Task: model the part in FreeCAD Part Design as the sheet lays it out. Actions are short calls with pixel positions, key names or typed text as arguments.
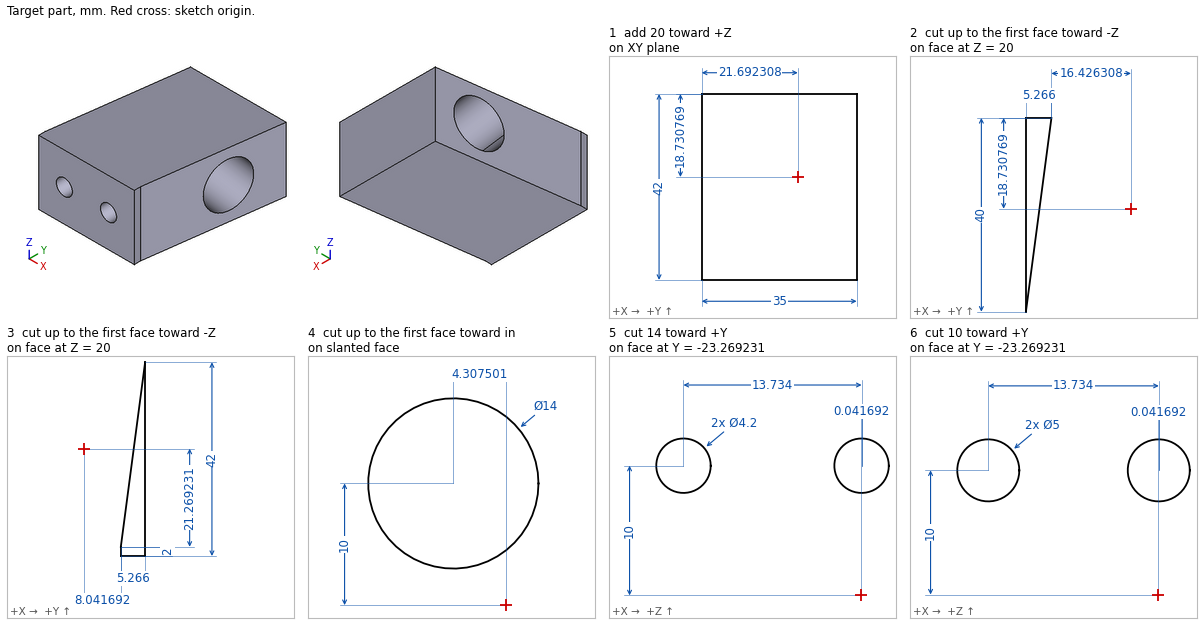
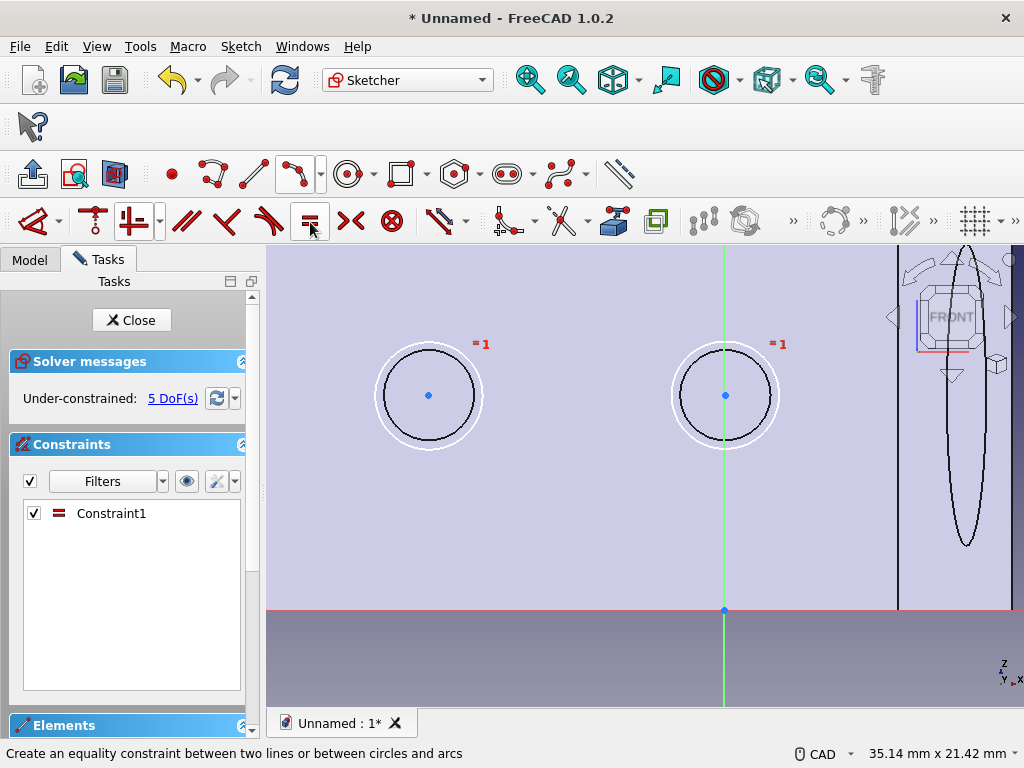
click(429, 396)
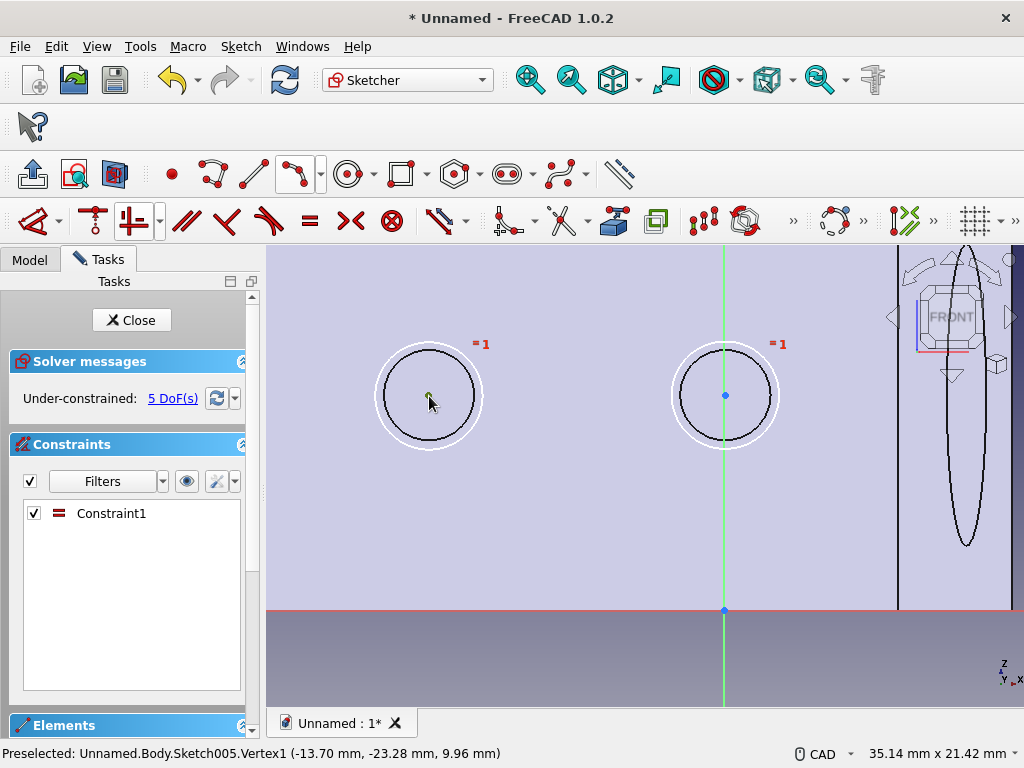
click(725, 395)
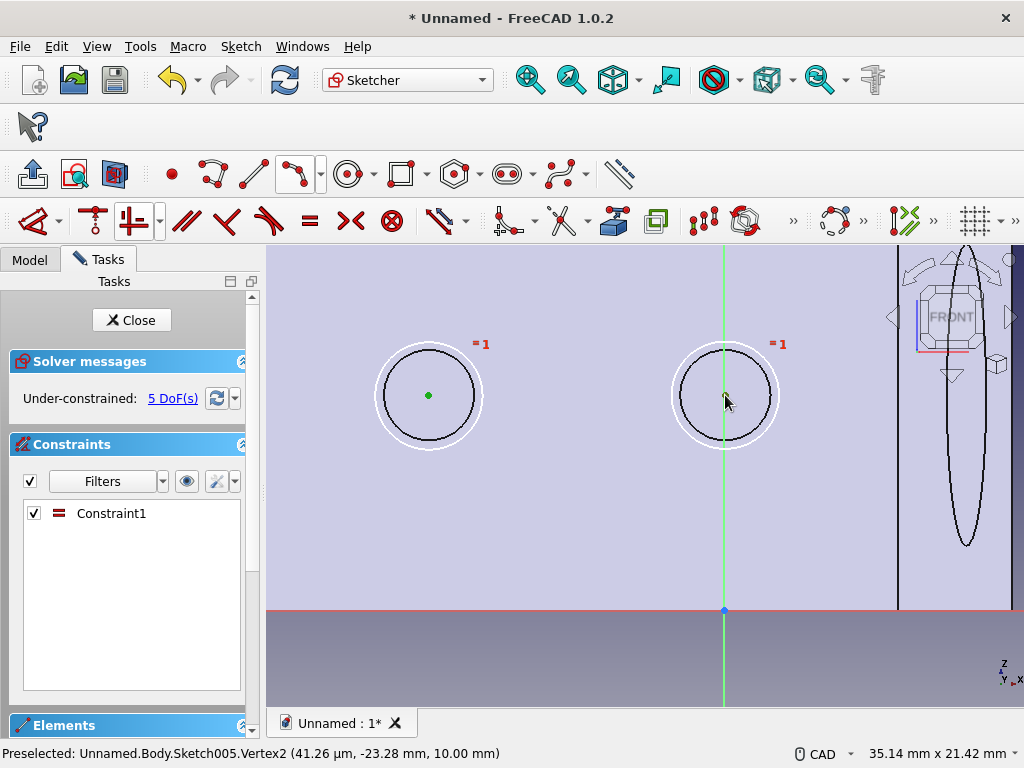
click(160, 222)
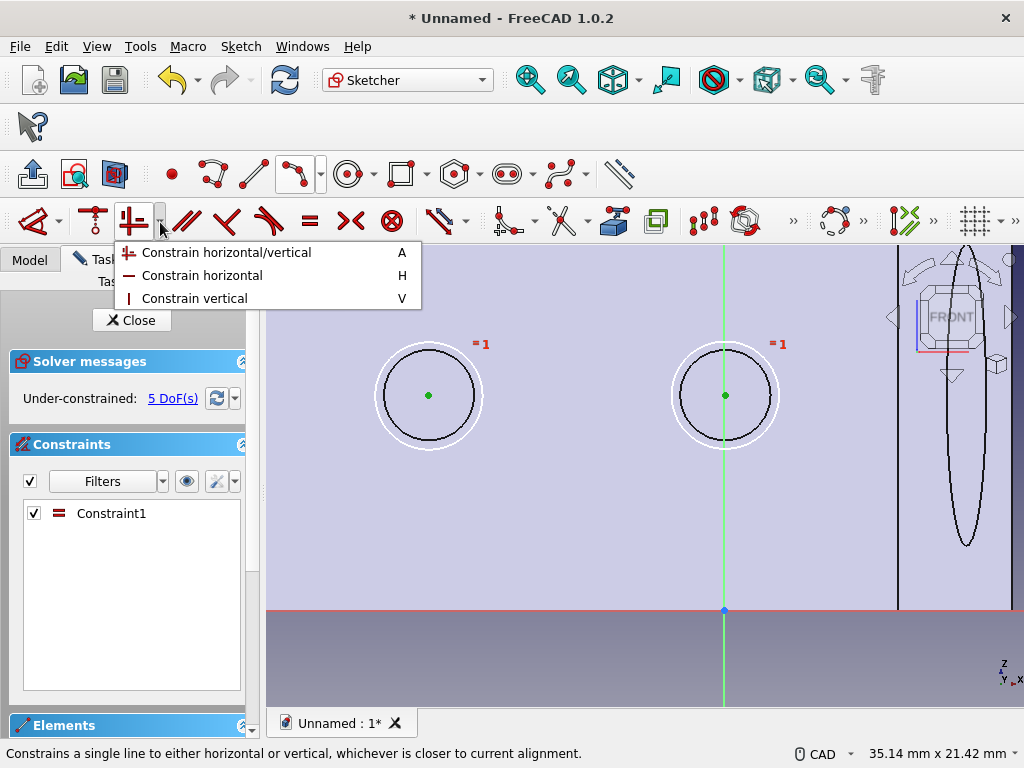
click(268, 276)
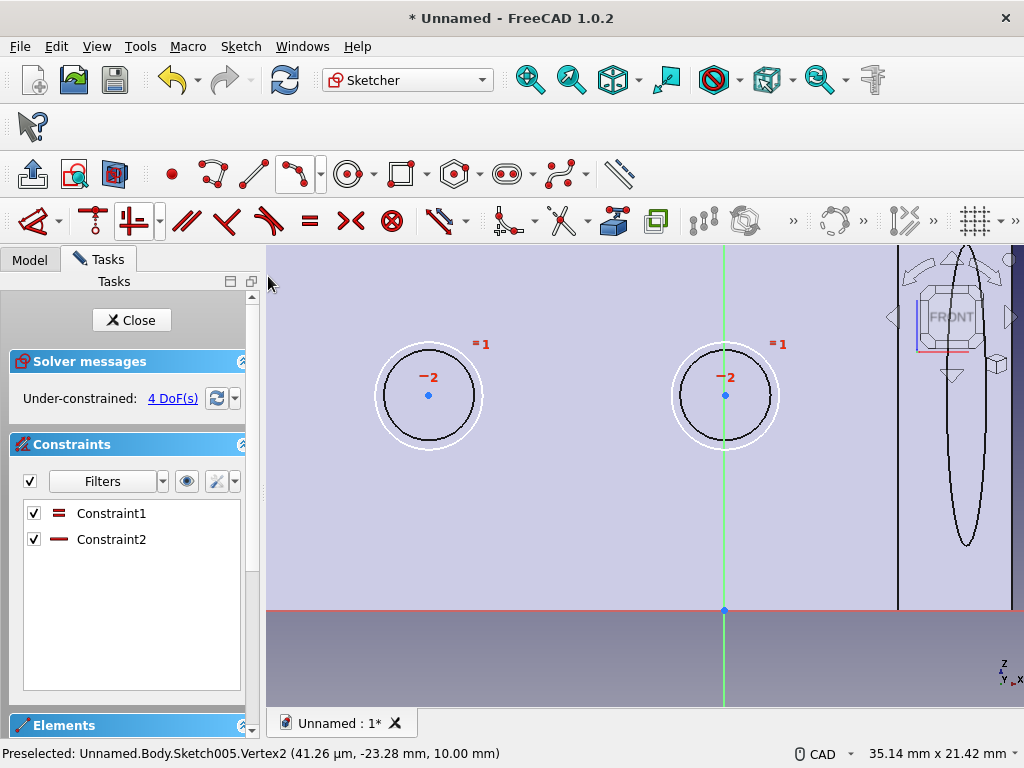
click(32, 222)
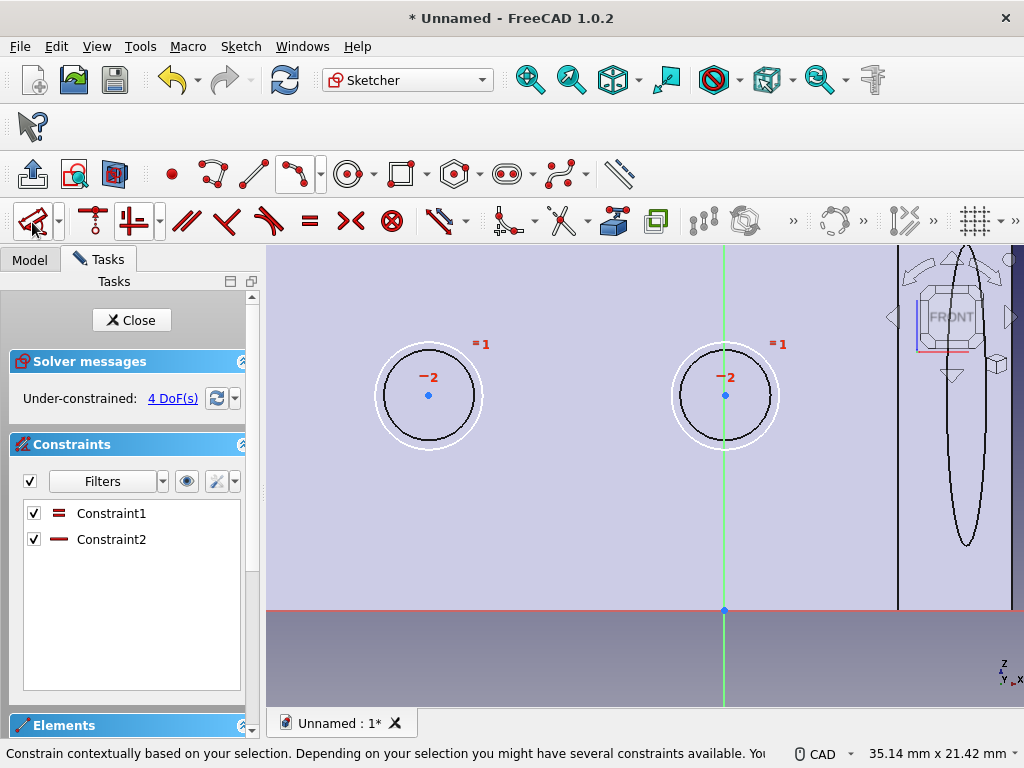
click(467, 358)
click(490, 335)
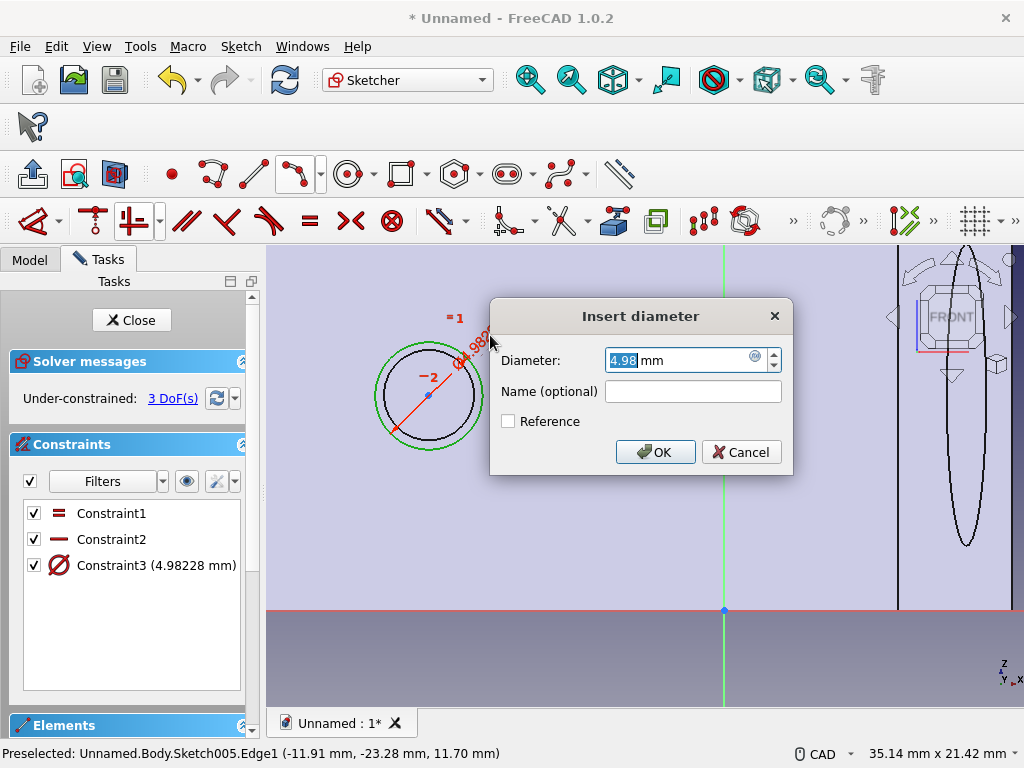
text(5)
key(Return)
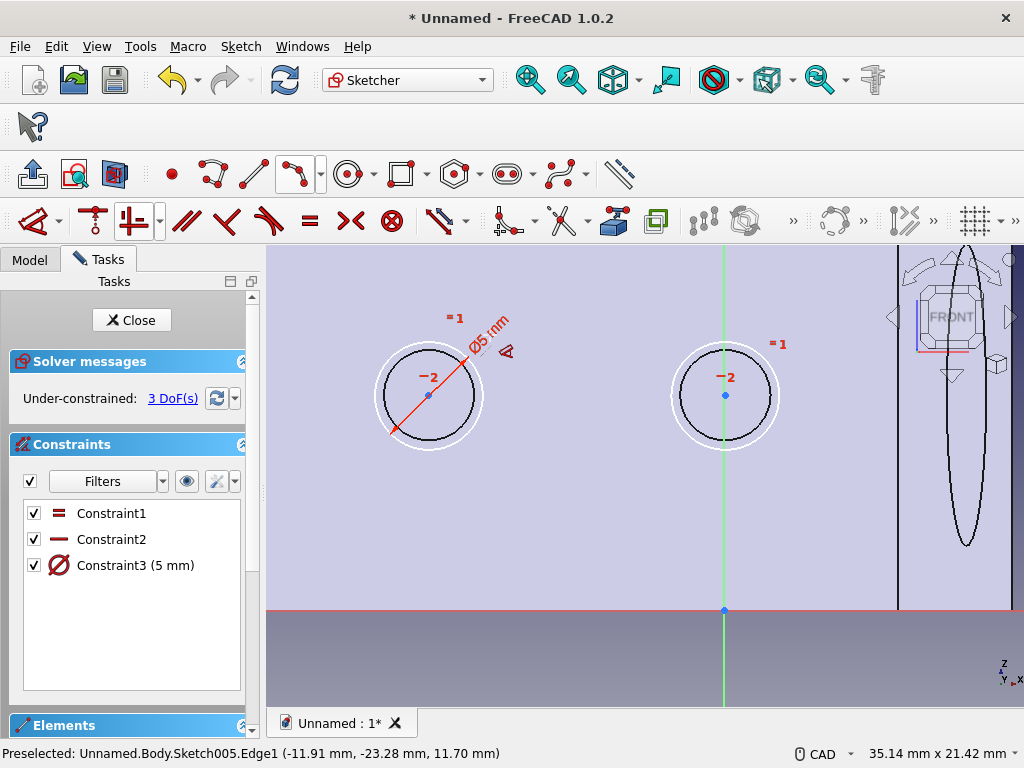
click(429, 396)
click(395, 503)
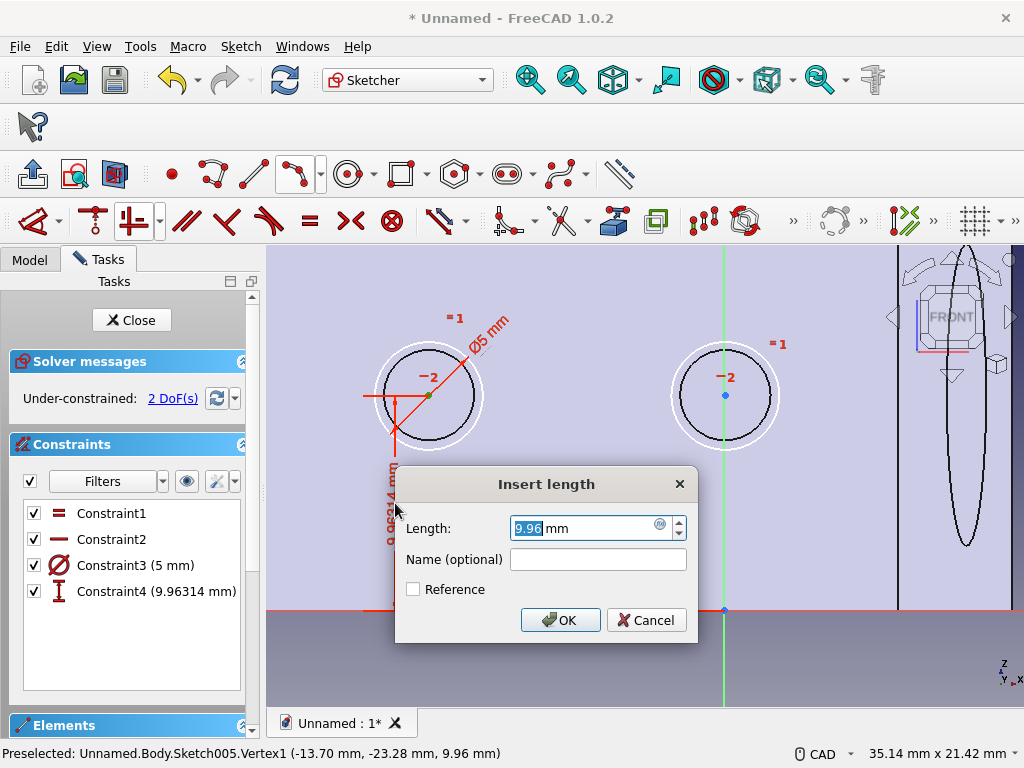
text(10)
key(Return)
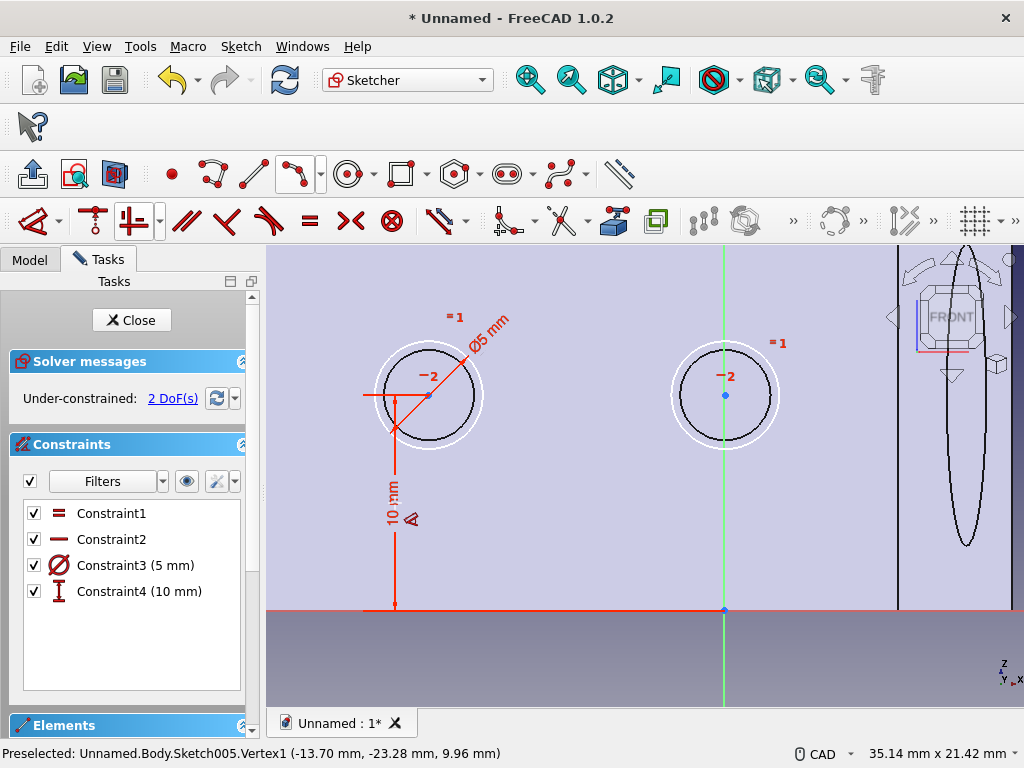
click(429, 395)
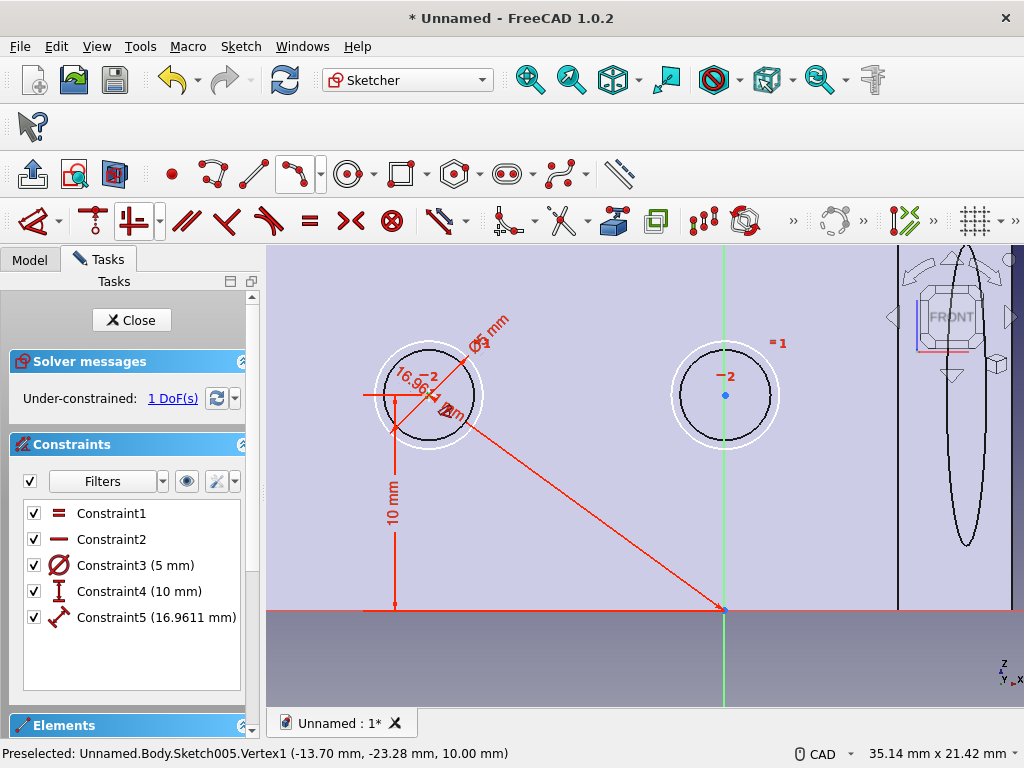
click(725, 395)
click(577, 361)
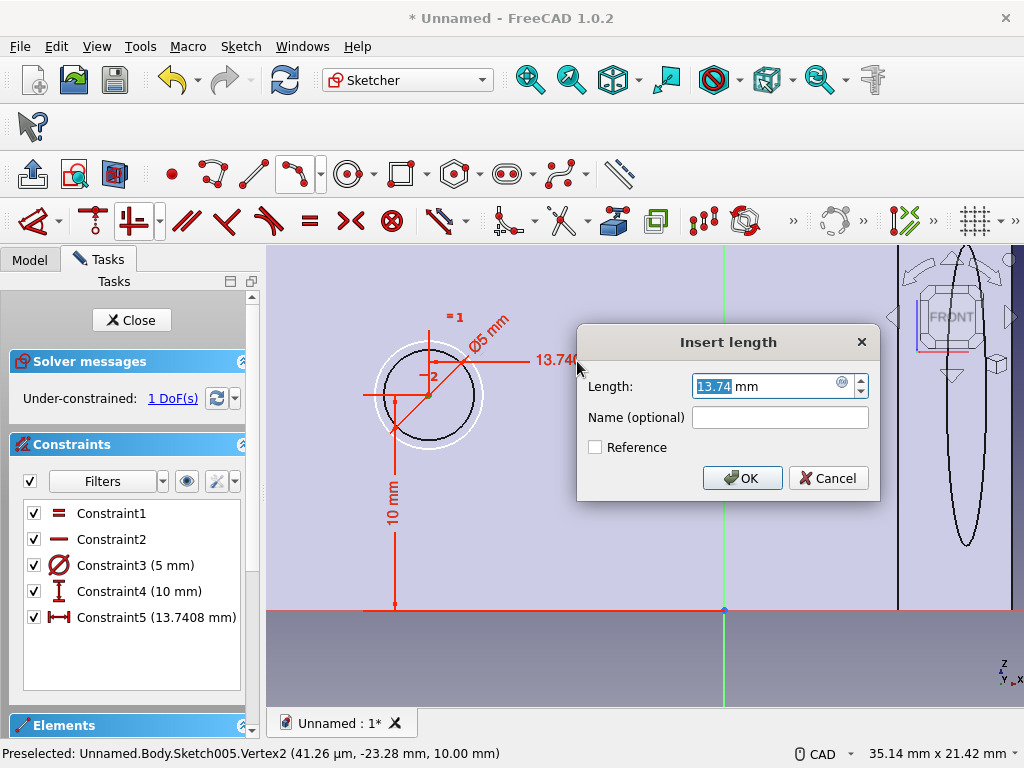
text(13.734)
key(Return)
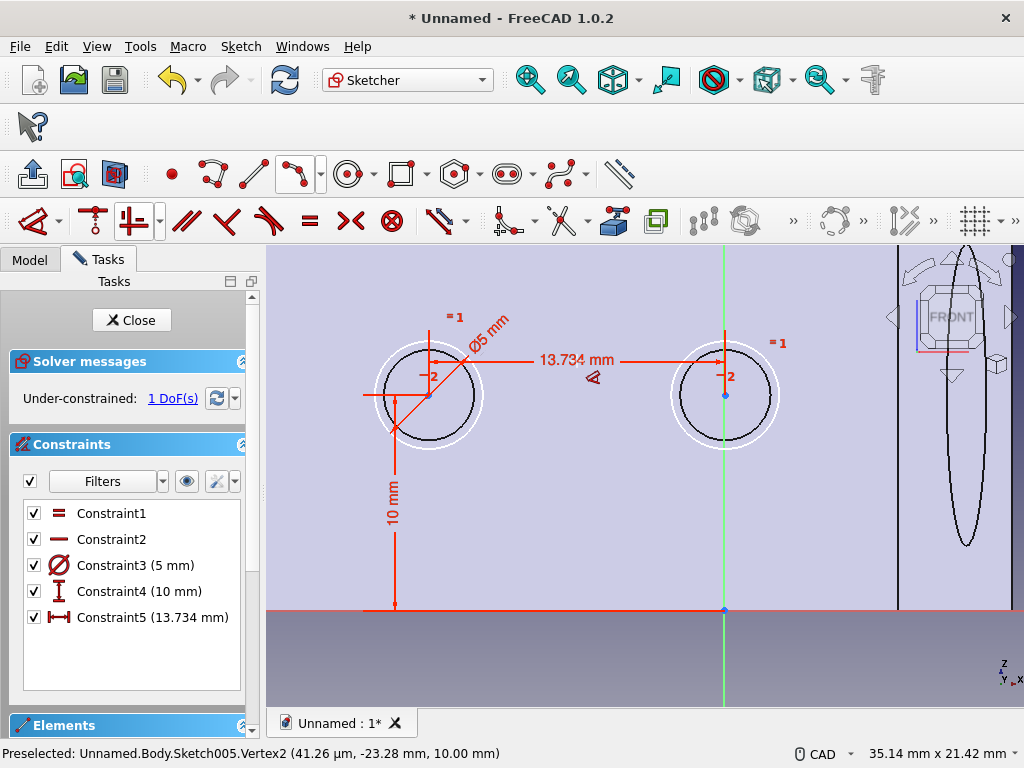
scroll(725, 395, up, 19)